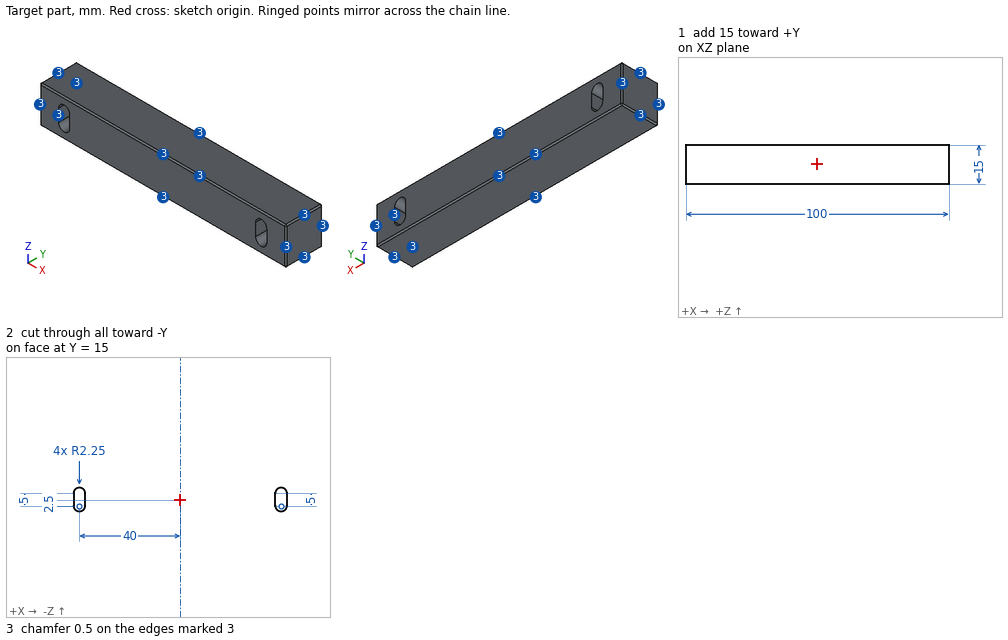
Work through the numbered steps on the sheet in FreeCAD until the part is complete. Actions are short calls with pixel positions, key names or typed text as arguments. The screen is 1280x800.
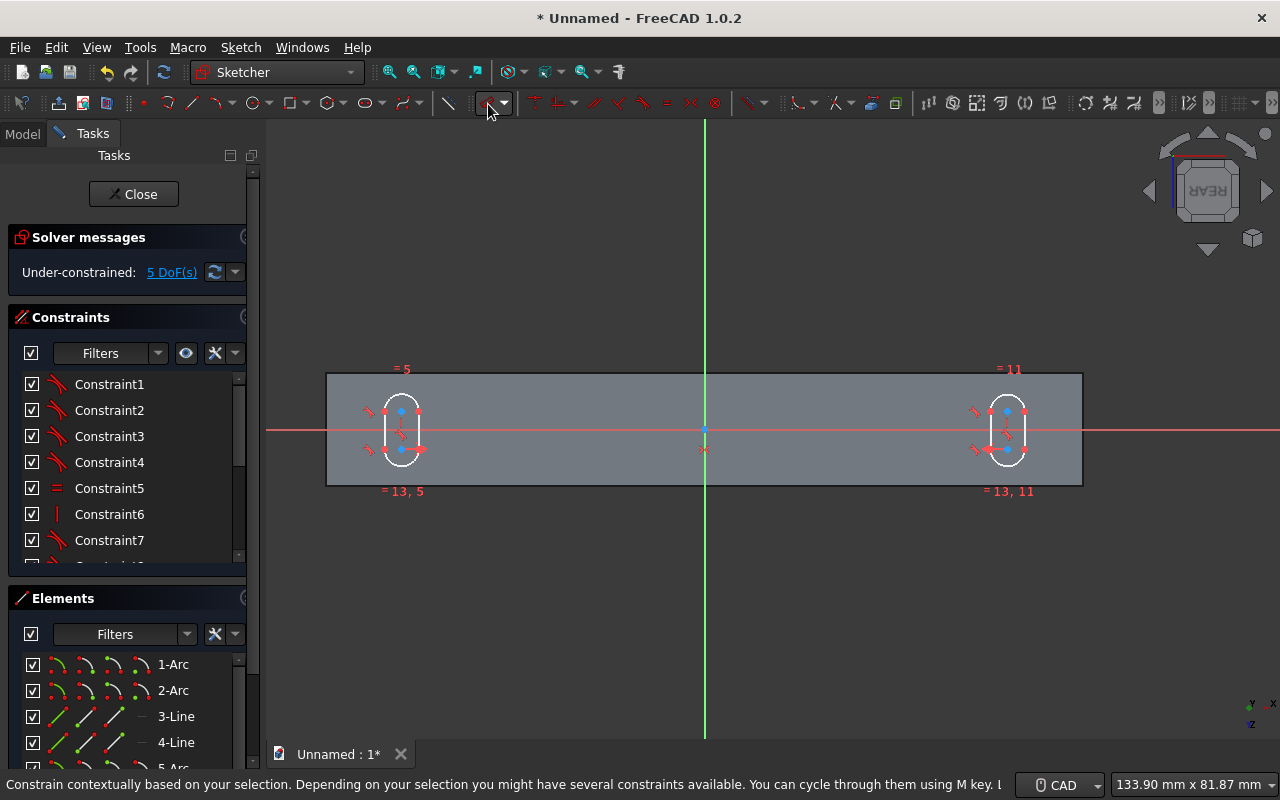
scroll(392, 463, up, 5)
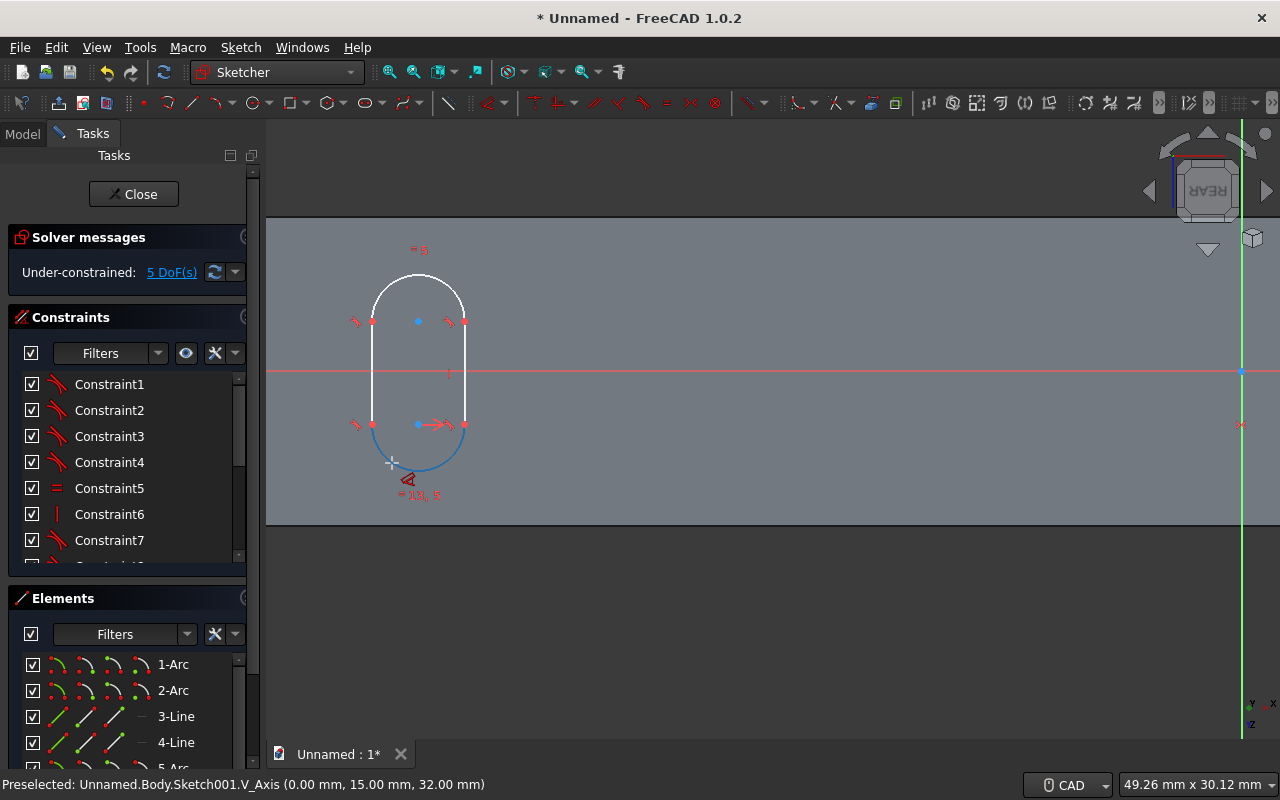
click(391, 462)
click(372, 488)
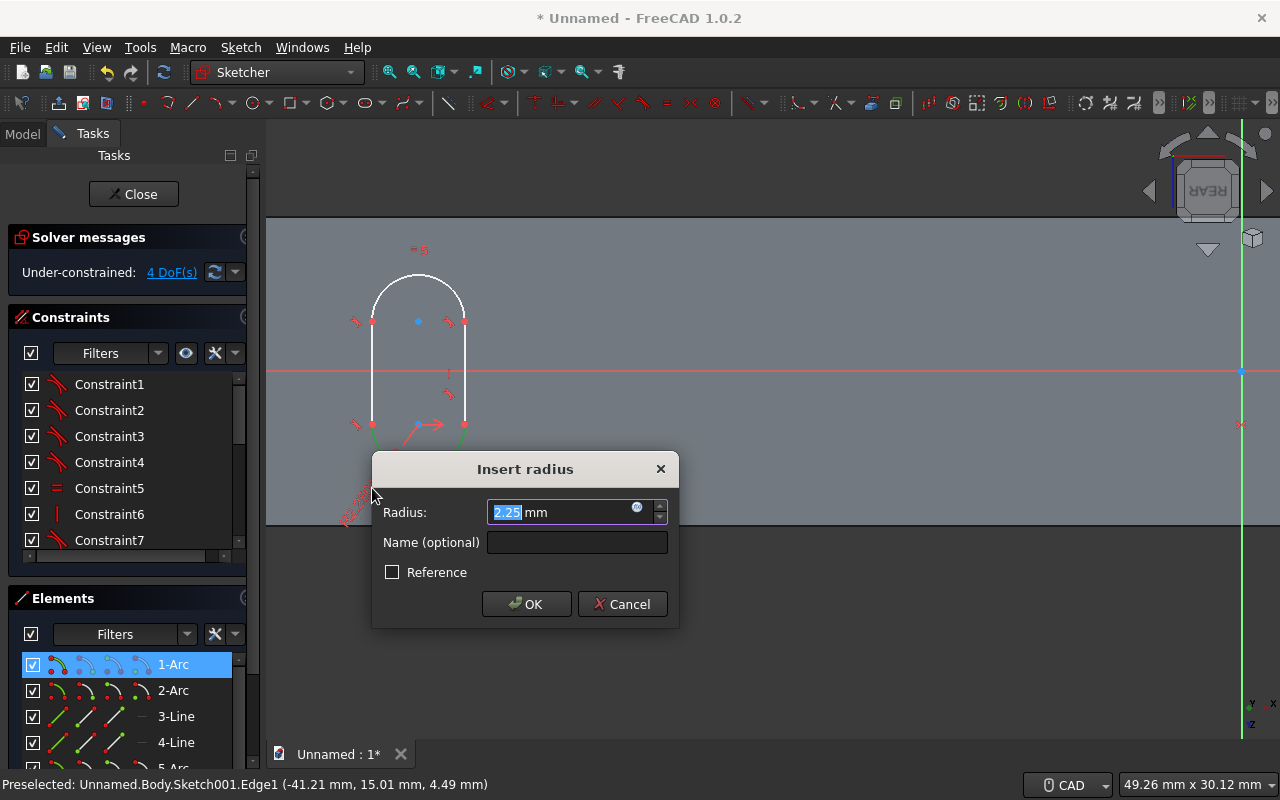
text(2.25)
key(Return)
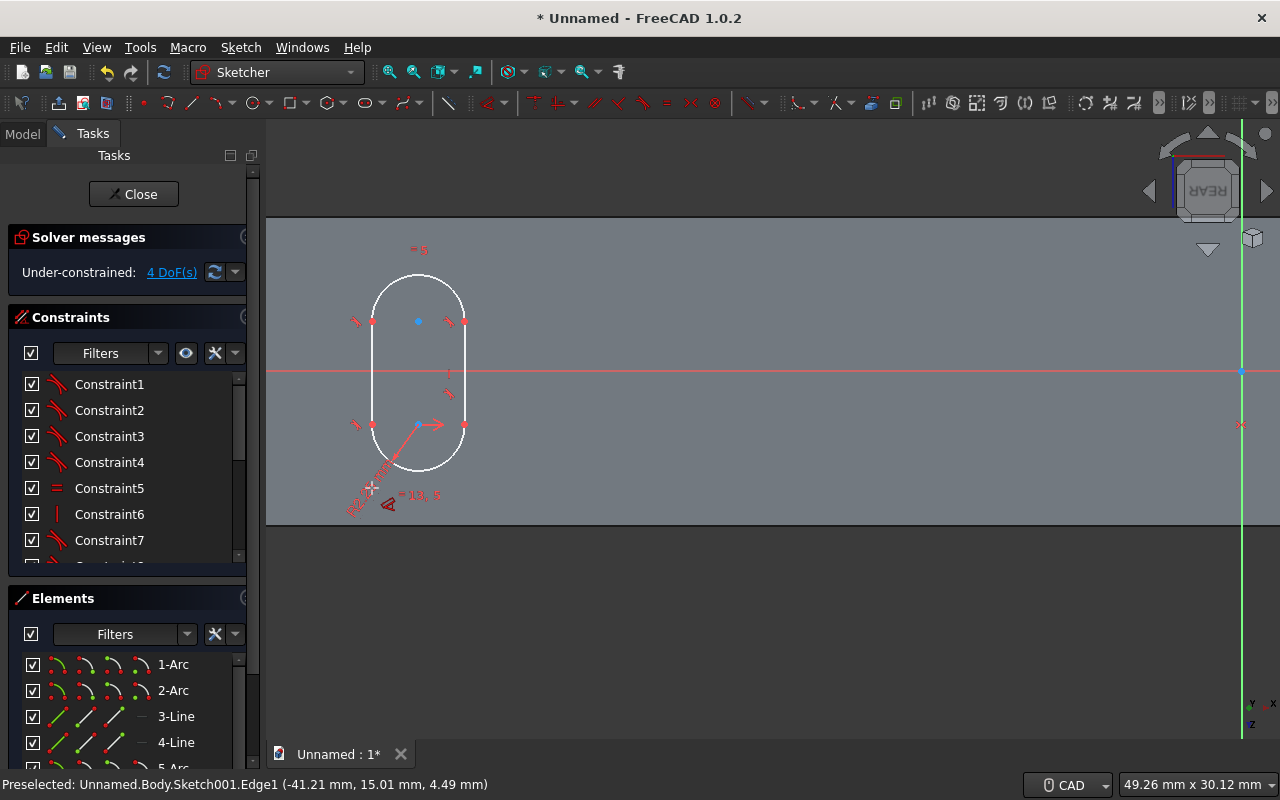
click(372, 394)
click(338, 349)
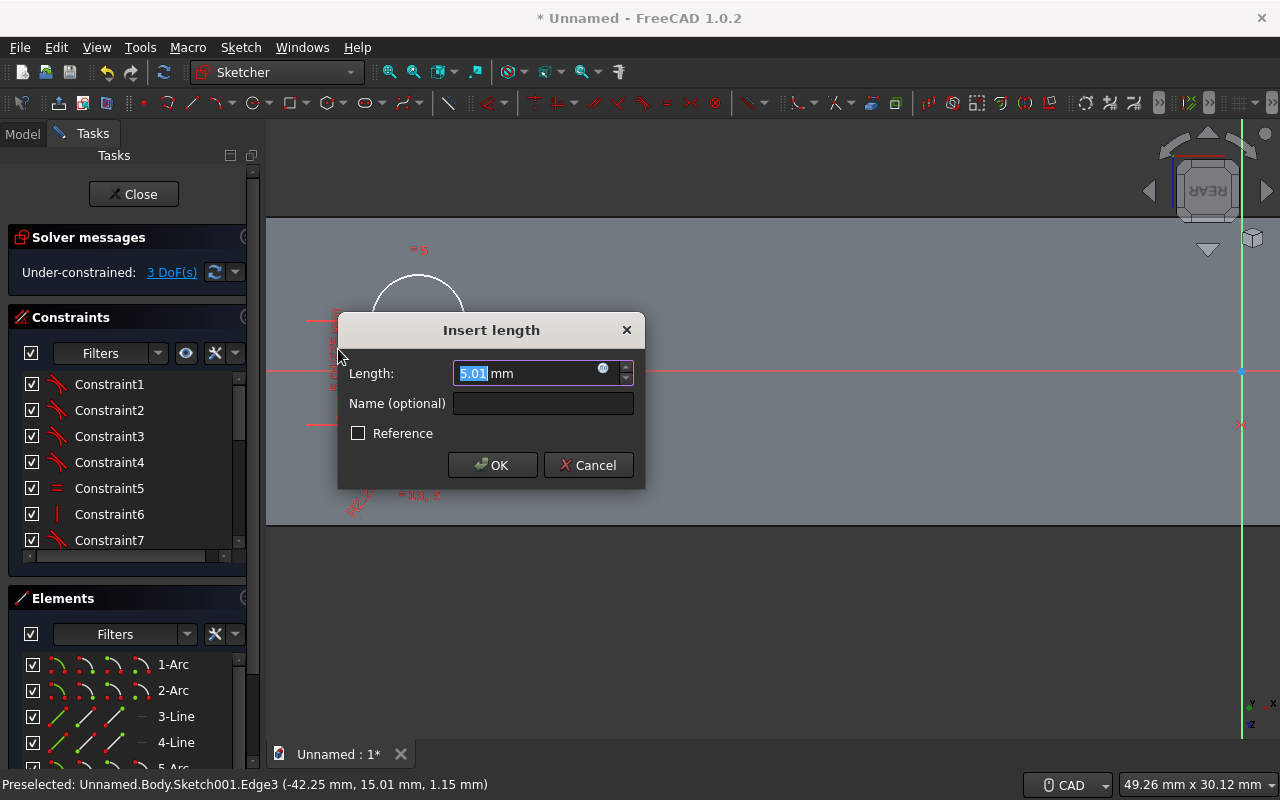
text(5)
key(Return)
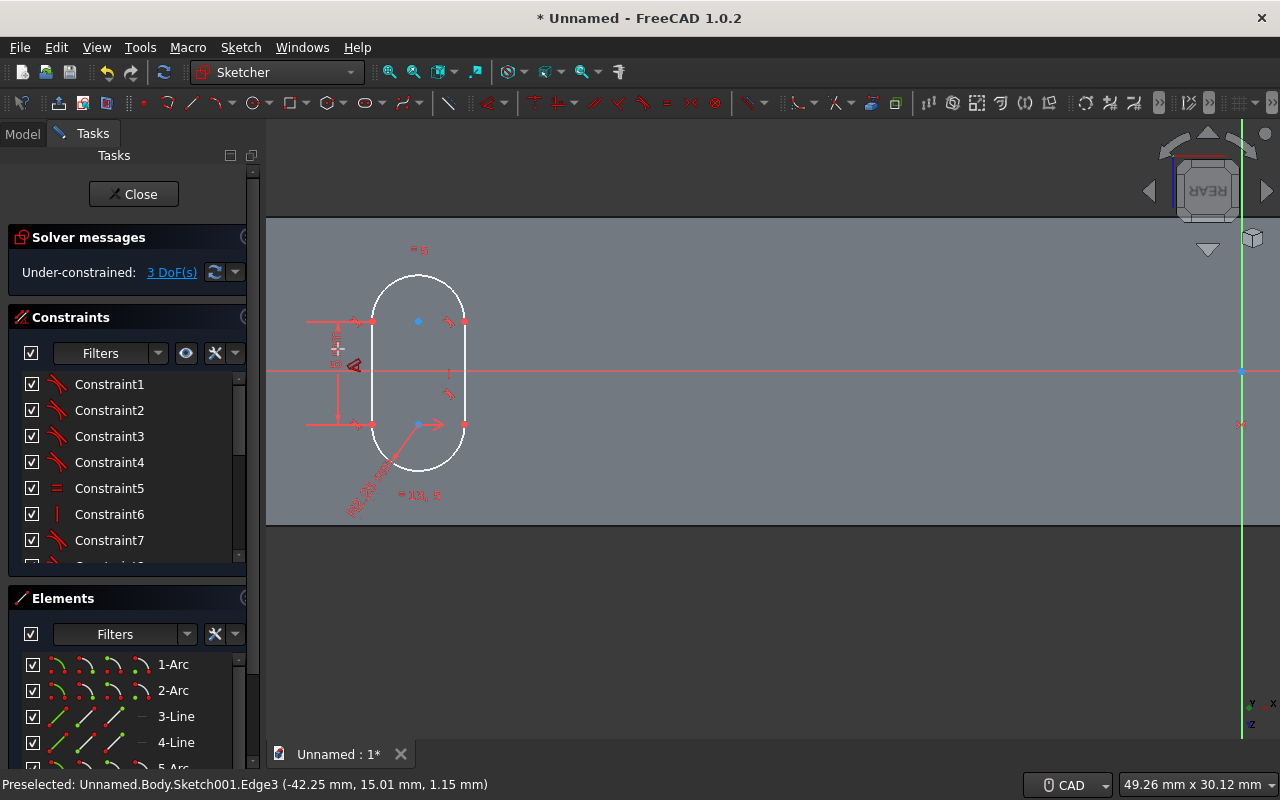
scroll(392, 463, down, 5)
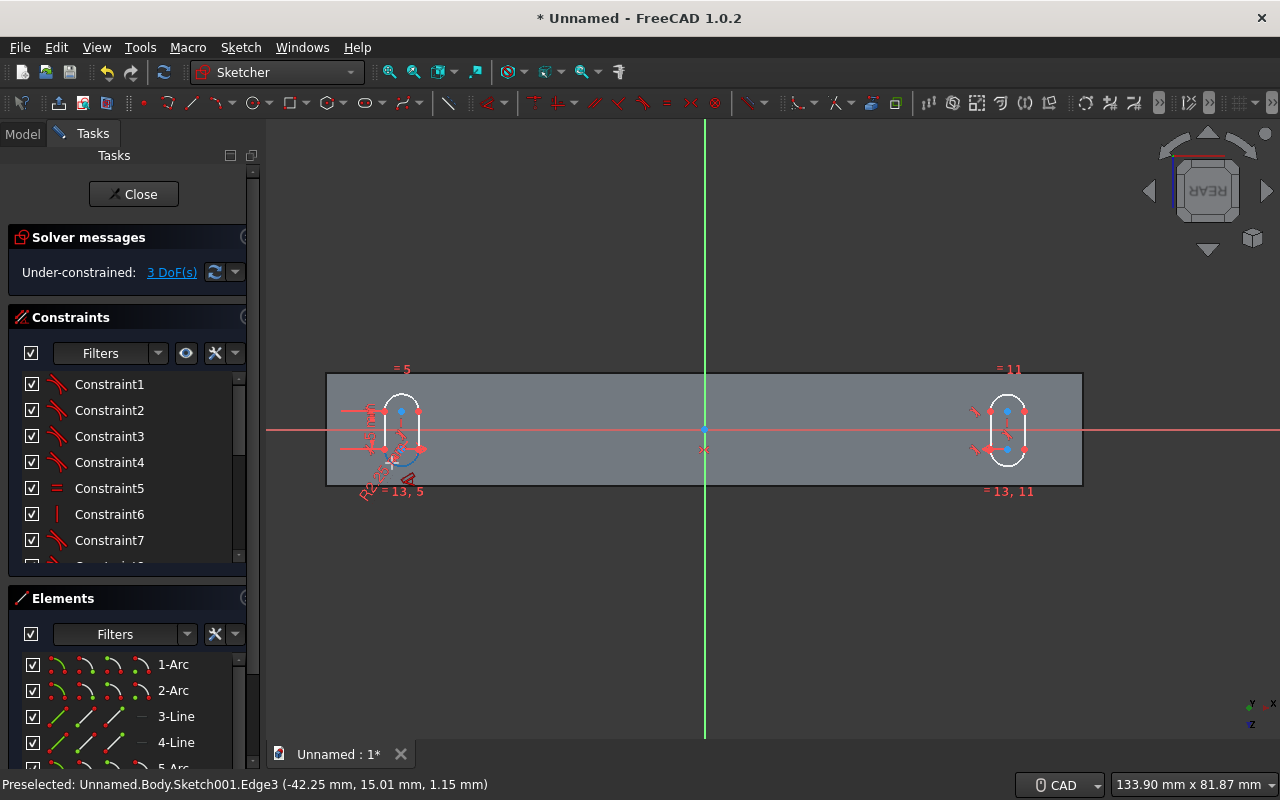
scroll(991, 438, up, 3)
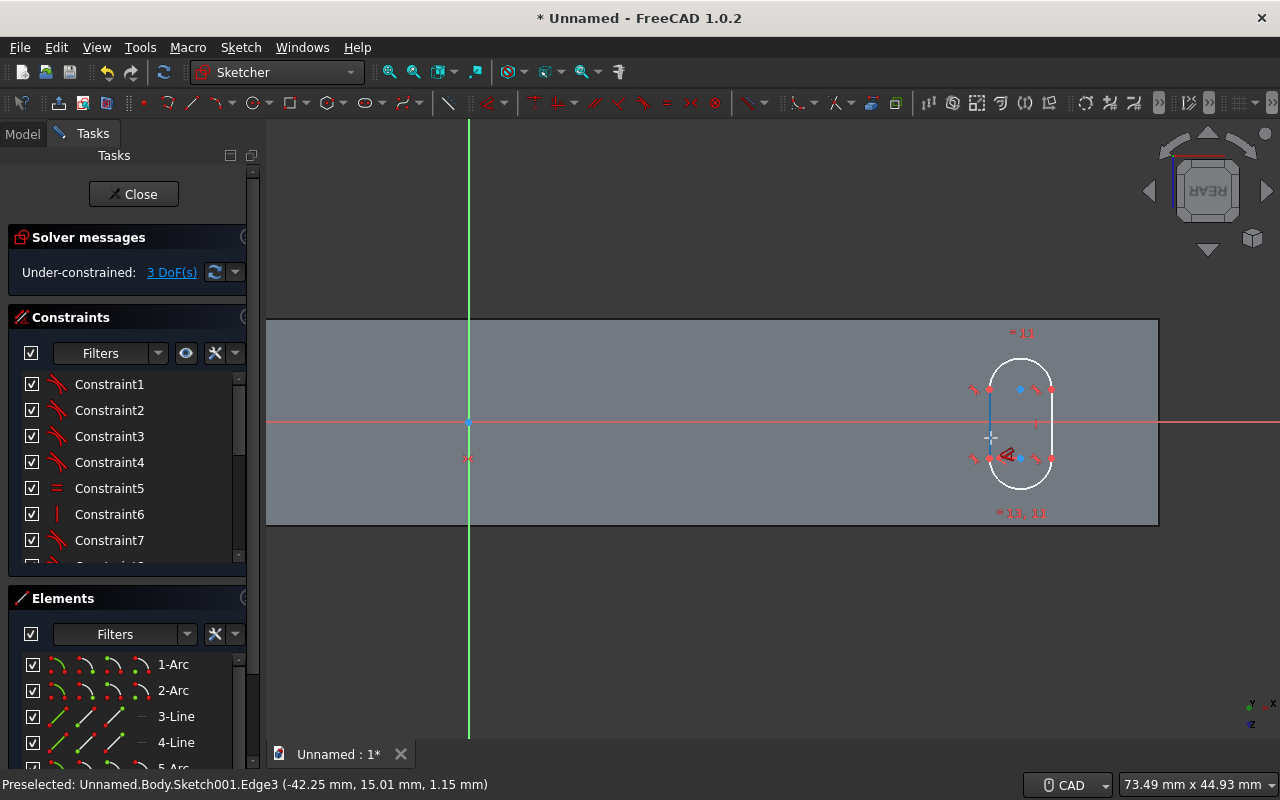
click(990, 438)
click(1024, 408)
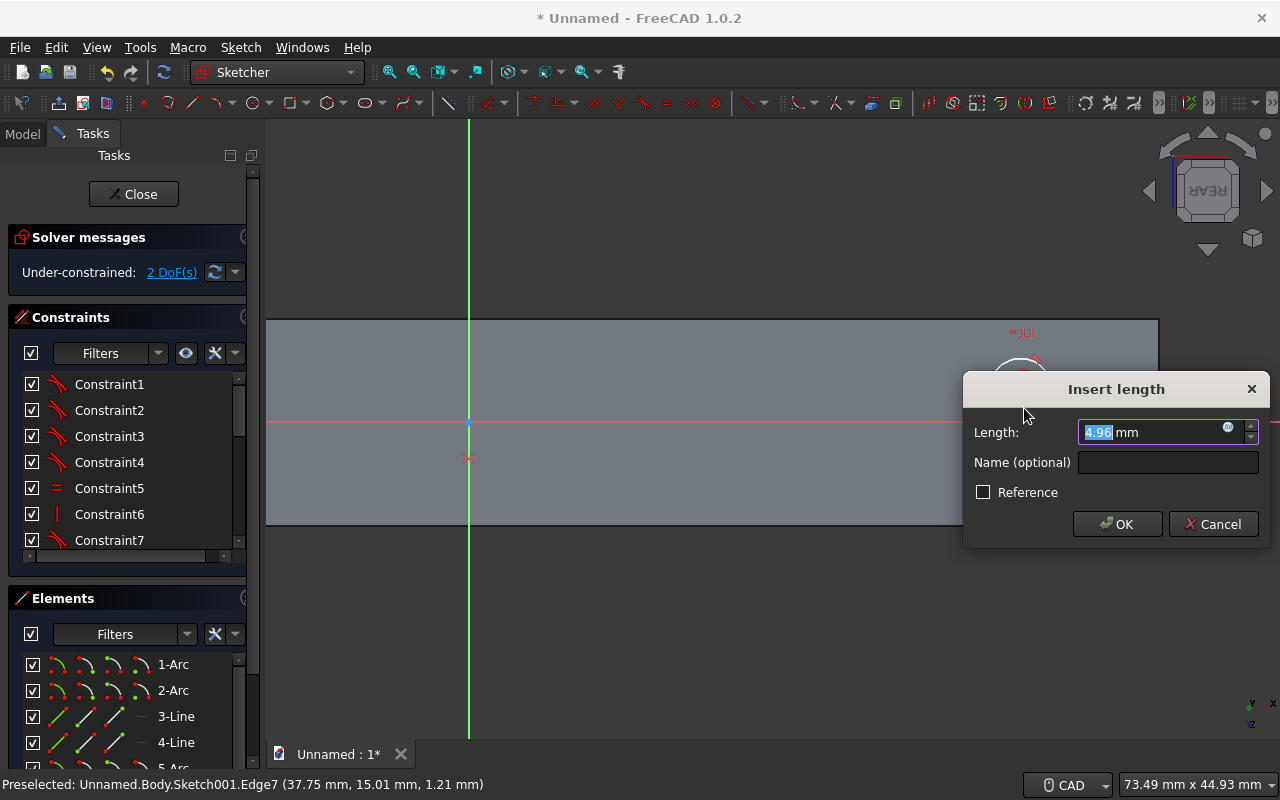
text(5)
key(Return)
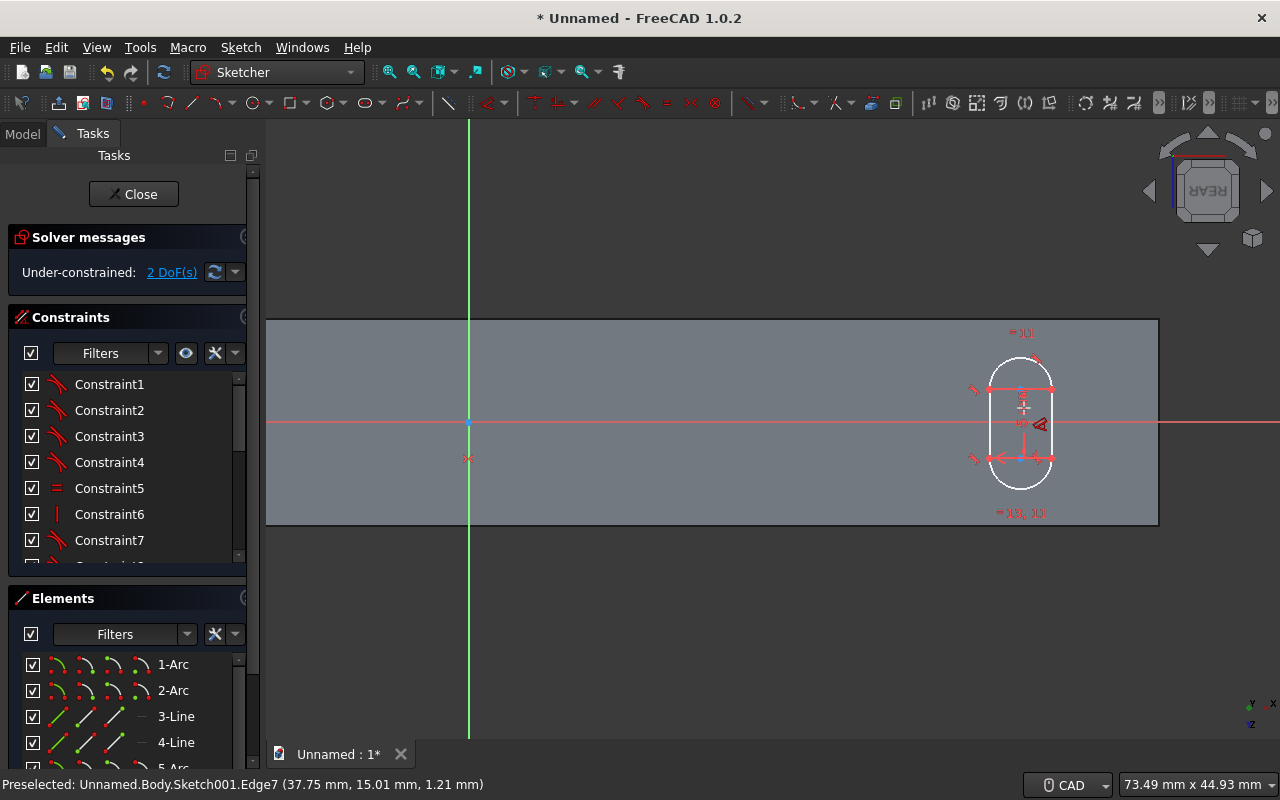
scroll(991, 437, down, 3)